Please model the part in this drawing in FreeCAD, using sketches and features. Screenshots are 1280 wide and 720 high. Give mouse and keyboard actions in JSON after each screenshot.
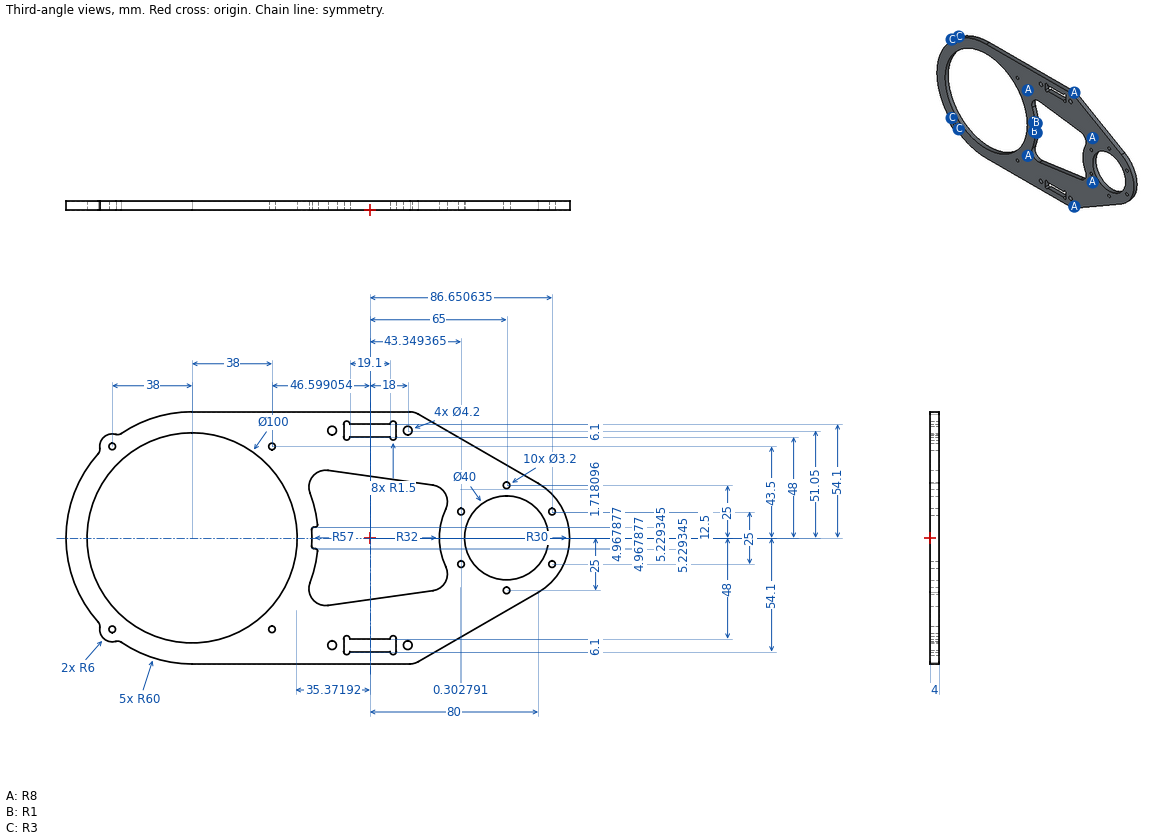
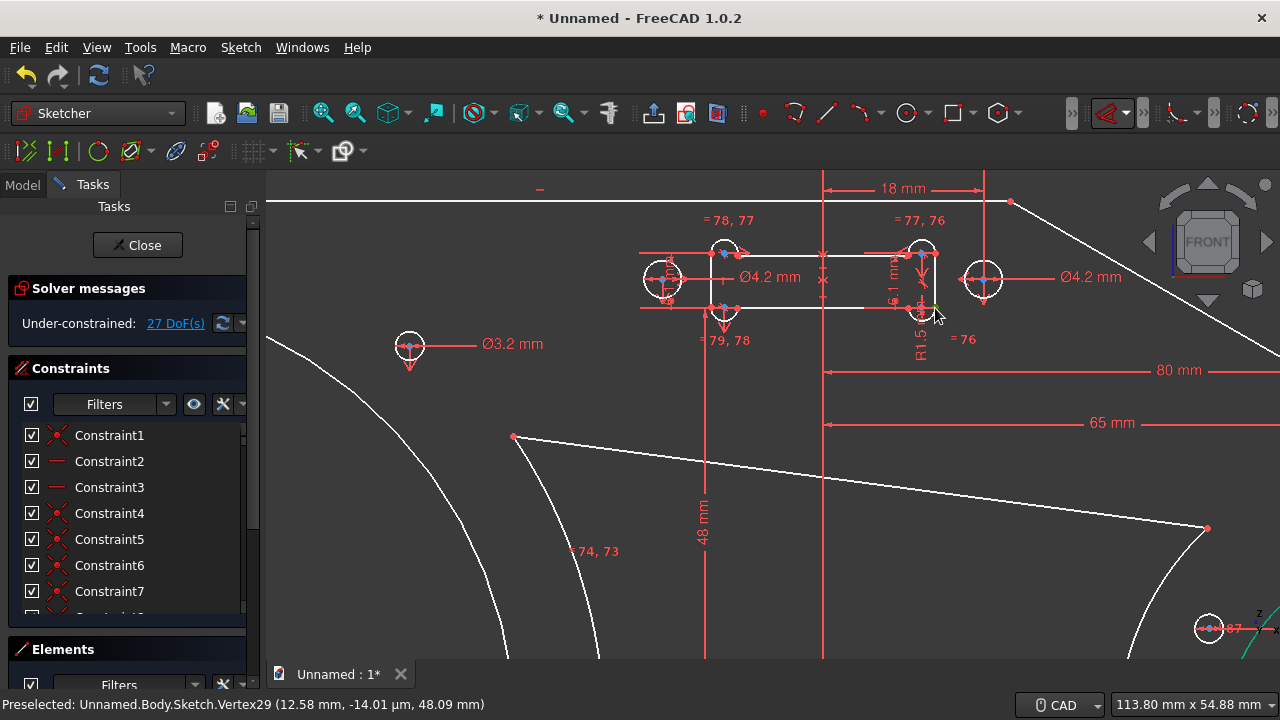
{"action": "left_click", "coordinate": [1128, 114]}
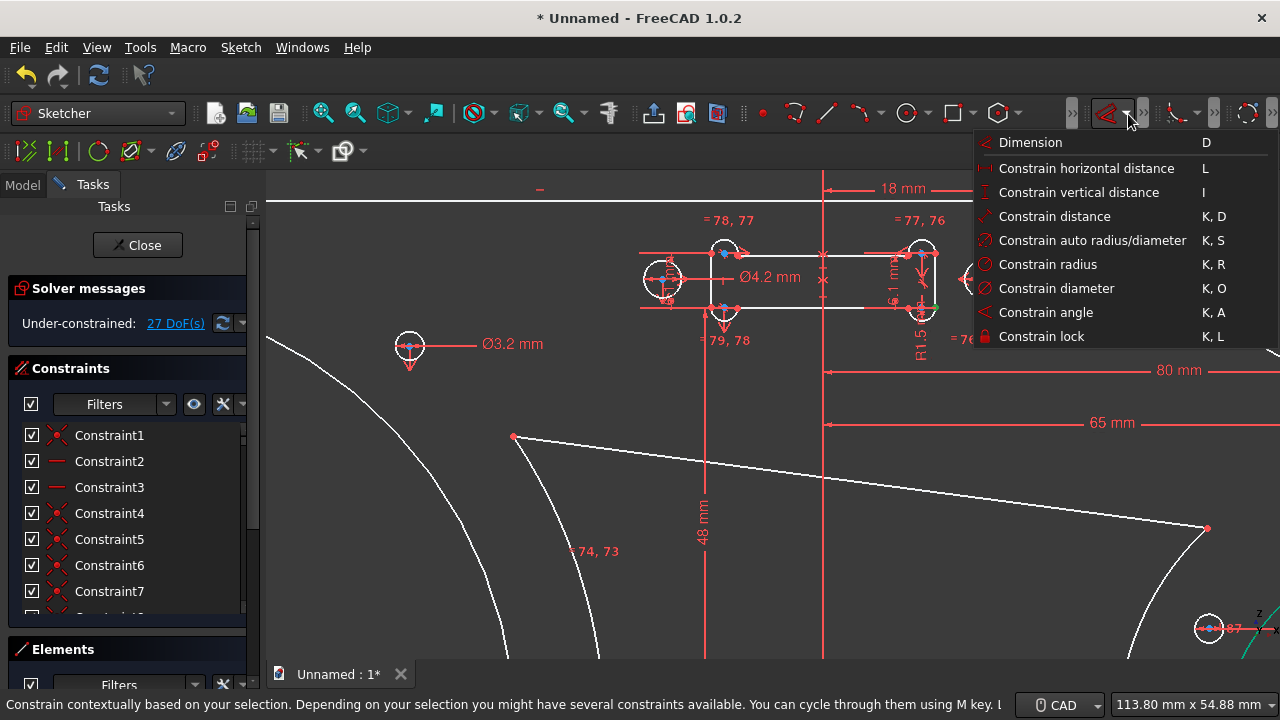
{"action": "left_click", "coordinate": [1126, 192]}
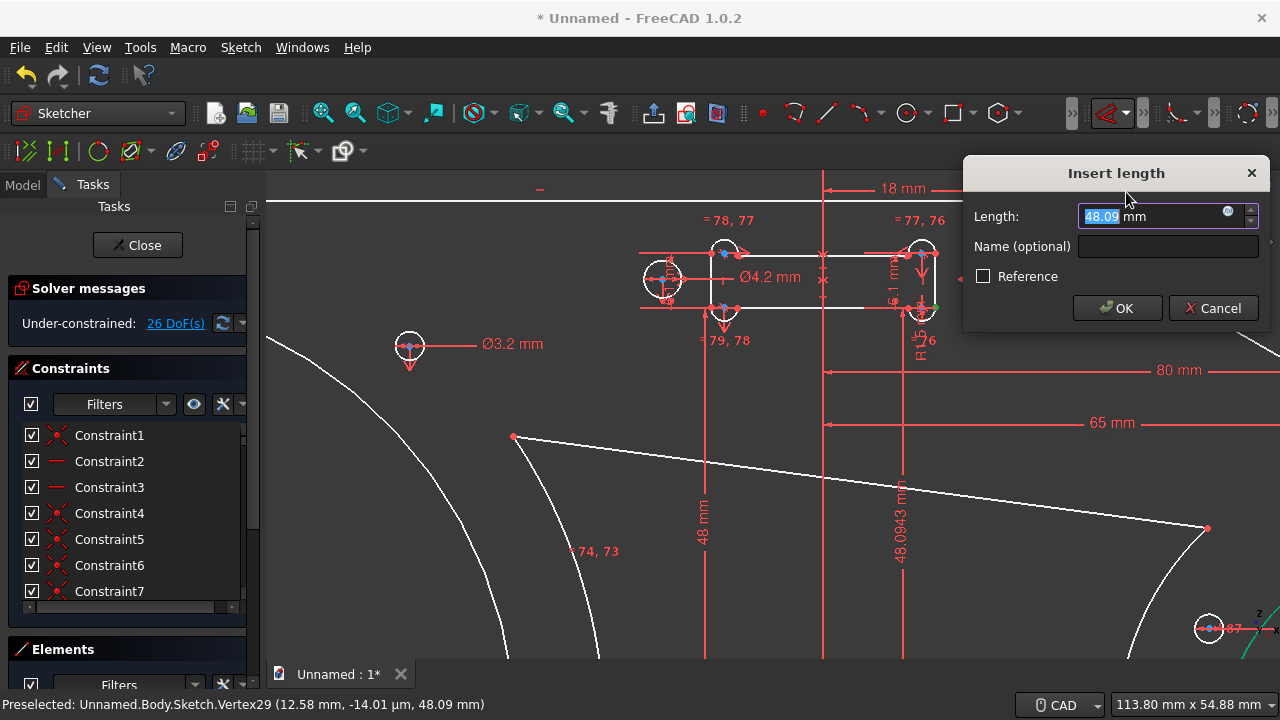
{"action": "type", "text": "48"}
{"action": "key", "text": "Return"}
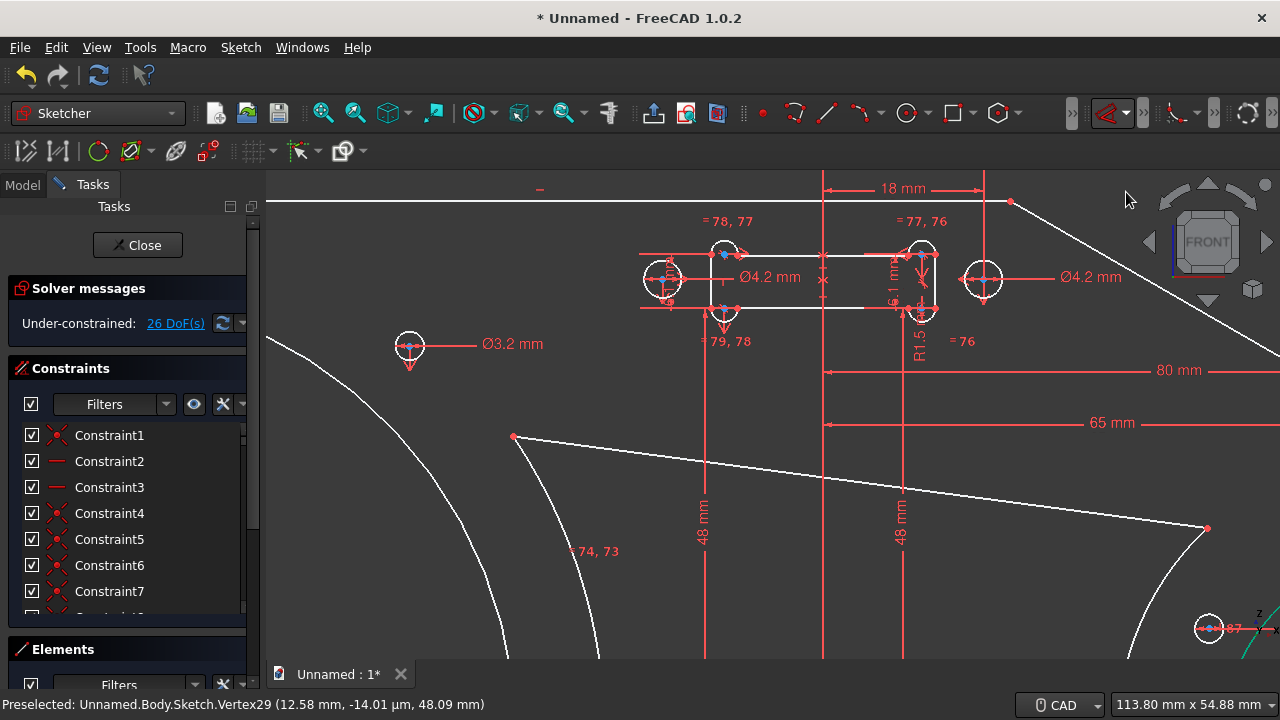
{"action": "scroll", "coordinate": [738, 309], "scroll_direction": "down", "scroll_amount": 7}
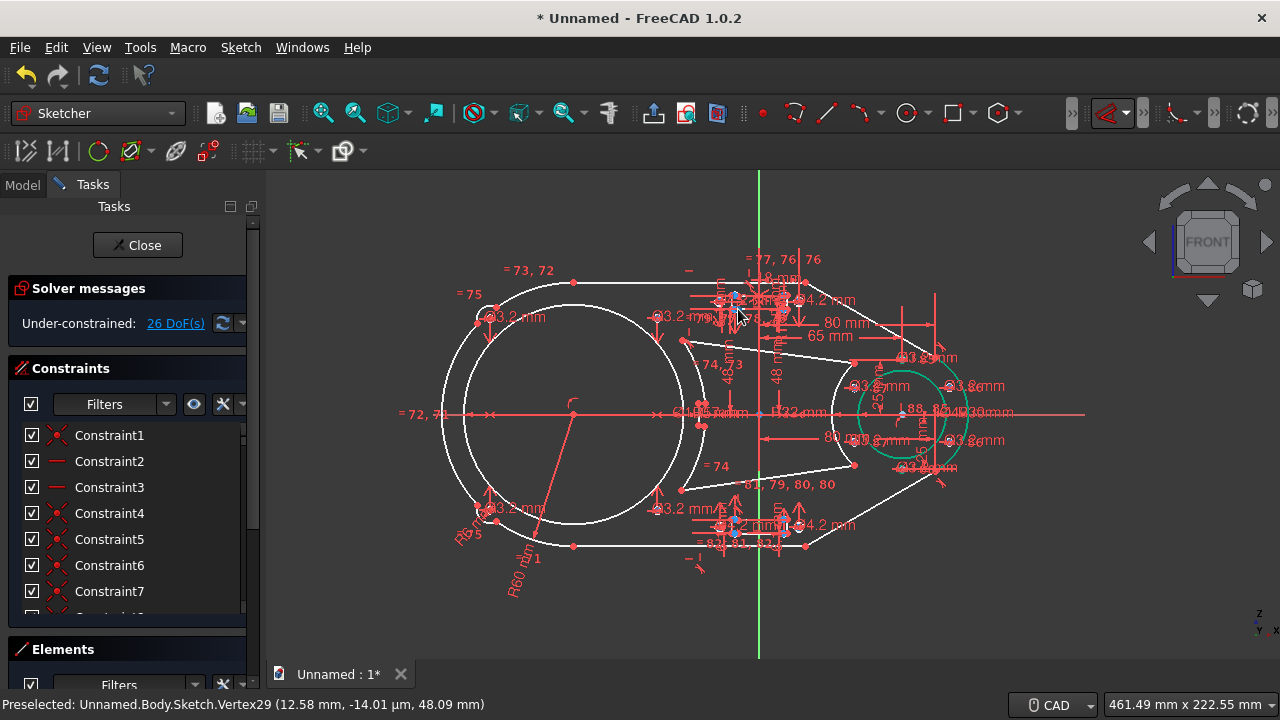
{"action": "scroll", "coordinate": [780, 520], "scroll_direction": "up", "scroll_amount": 7}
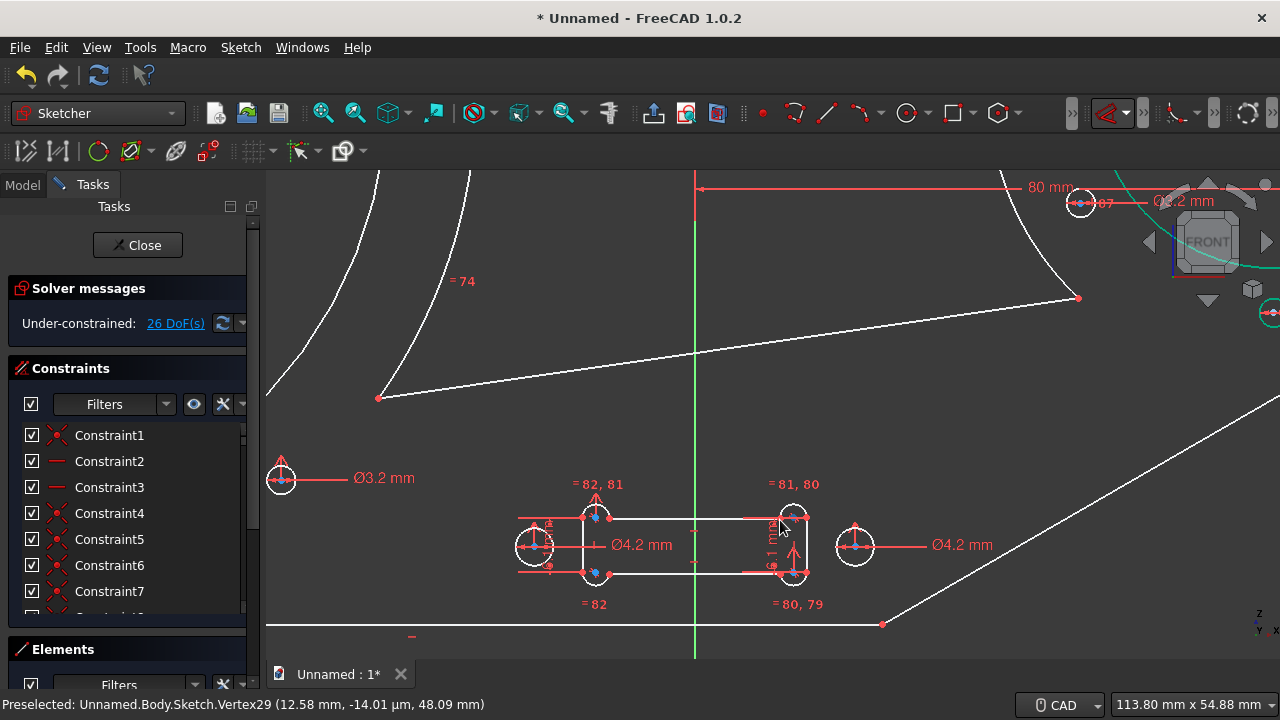
{"action": "left_click", "coordinate": [780, 519]}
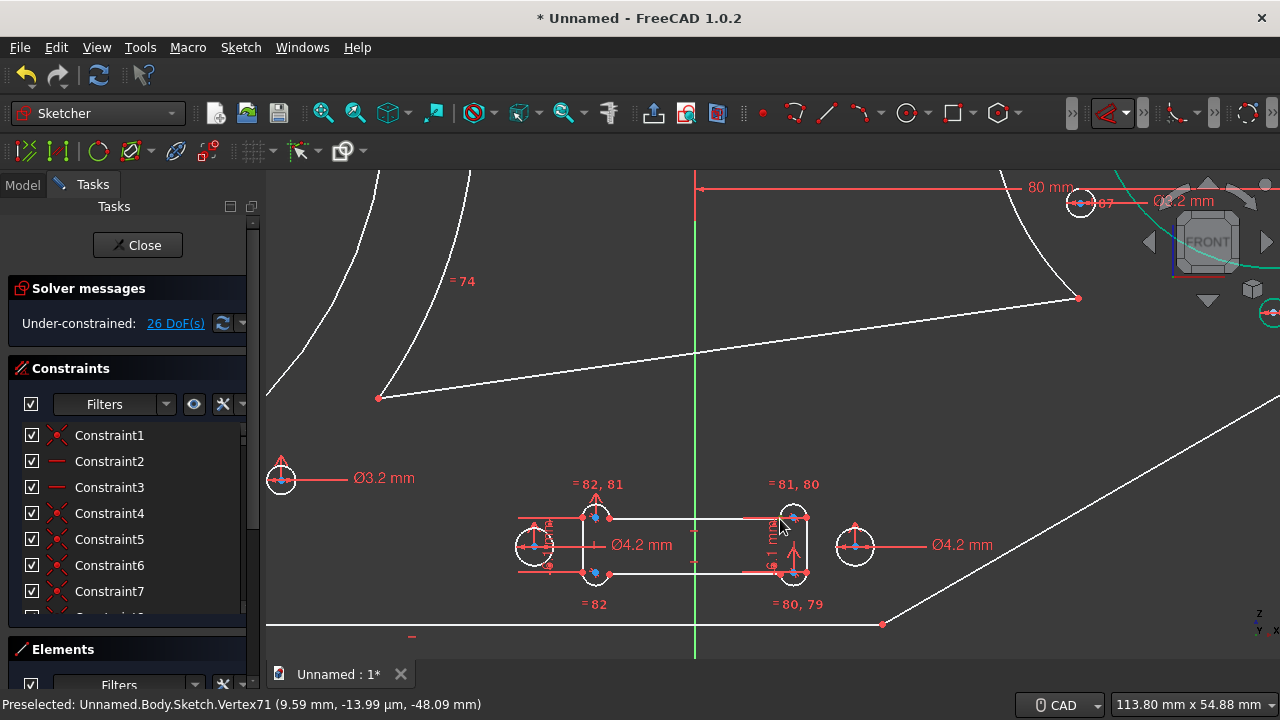
{"action": "key", "text": "i"}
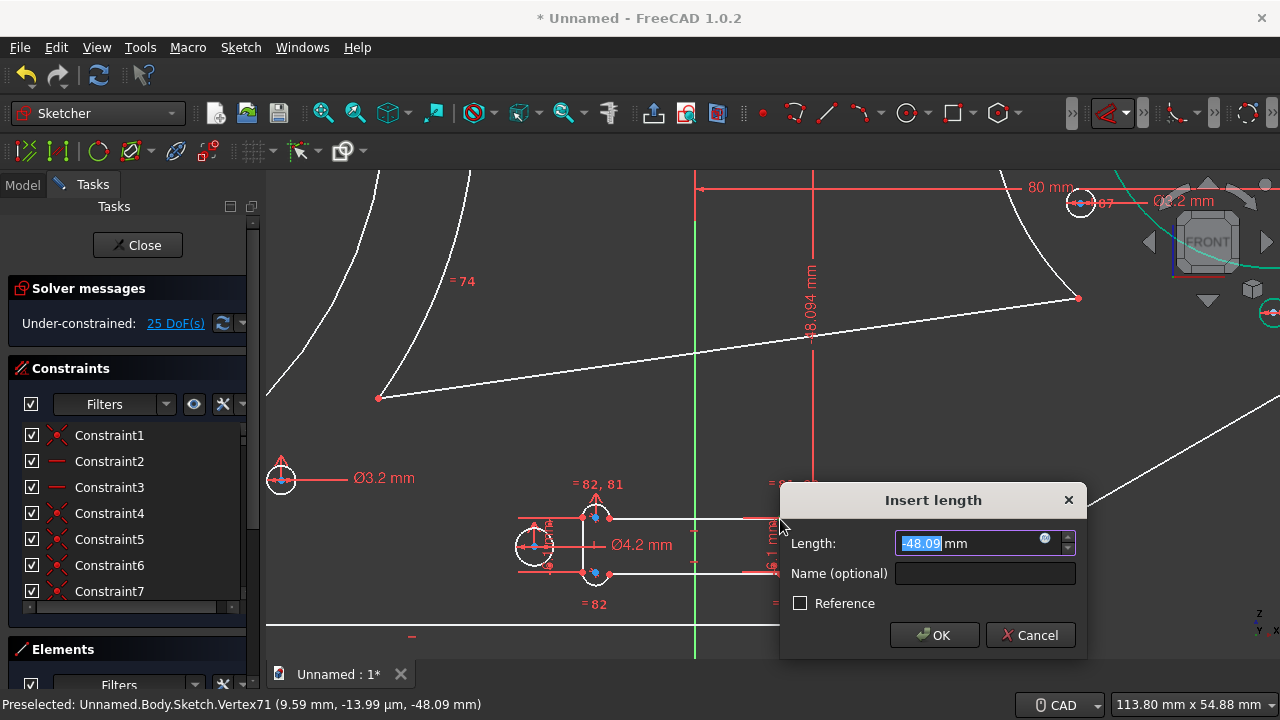
{"action": "type", "text": "-48"}
{"action": "key", "text": "Return"}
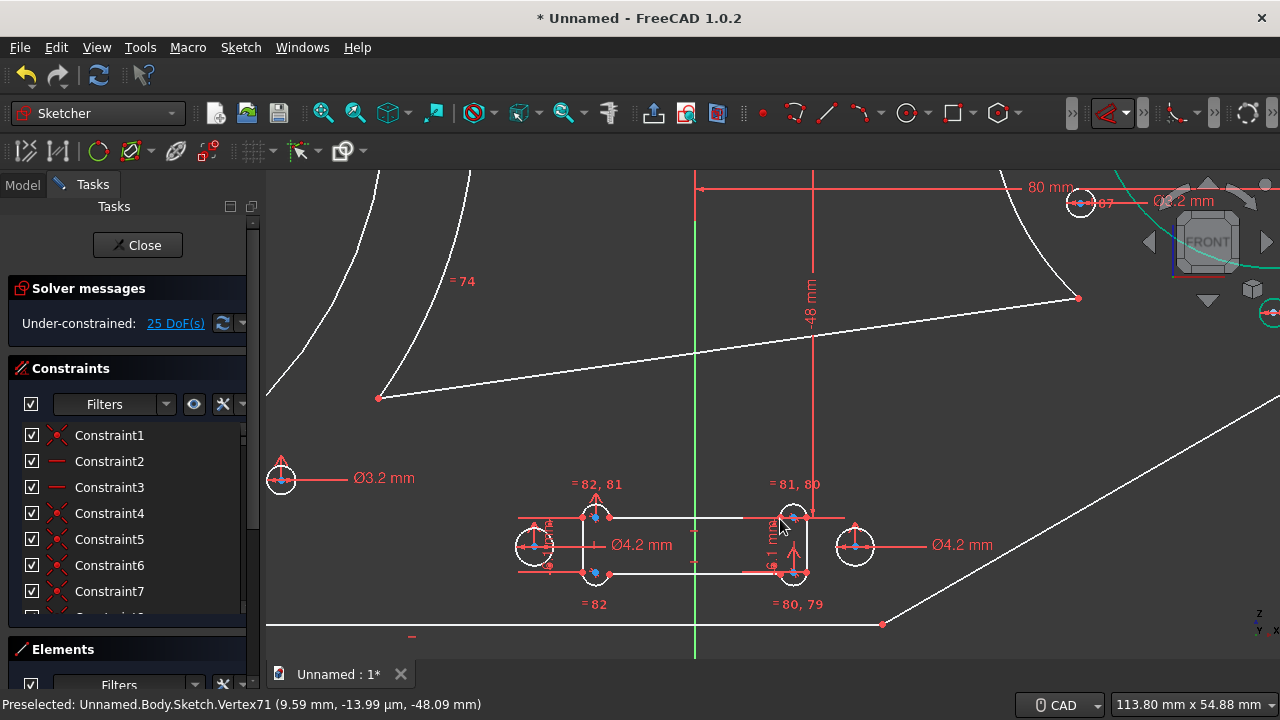
{"action": "scroll", "coordinate": [780, 521], "scroll_direction": "down", "scroll_amount": 7}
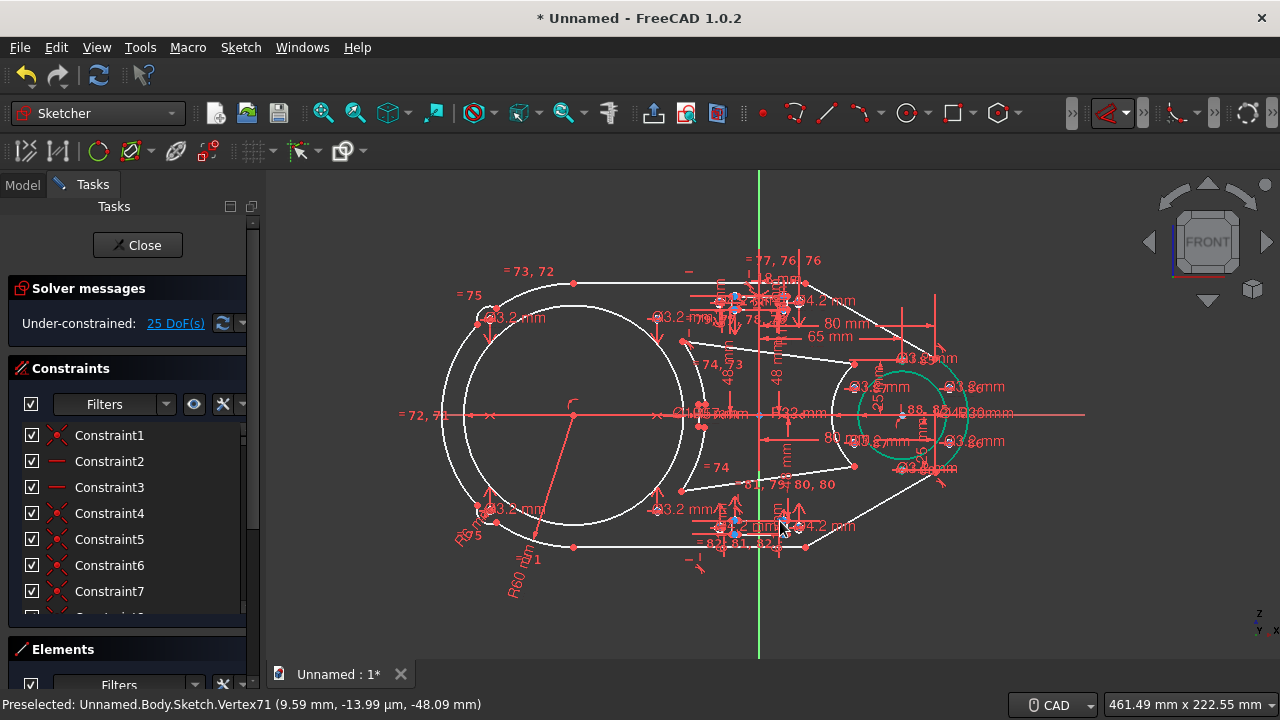
{"action": "left_click", "coordinate": [574, 283]}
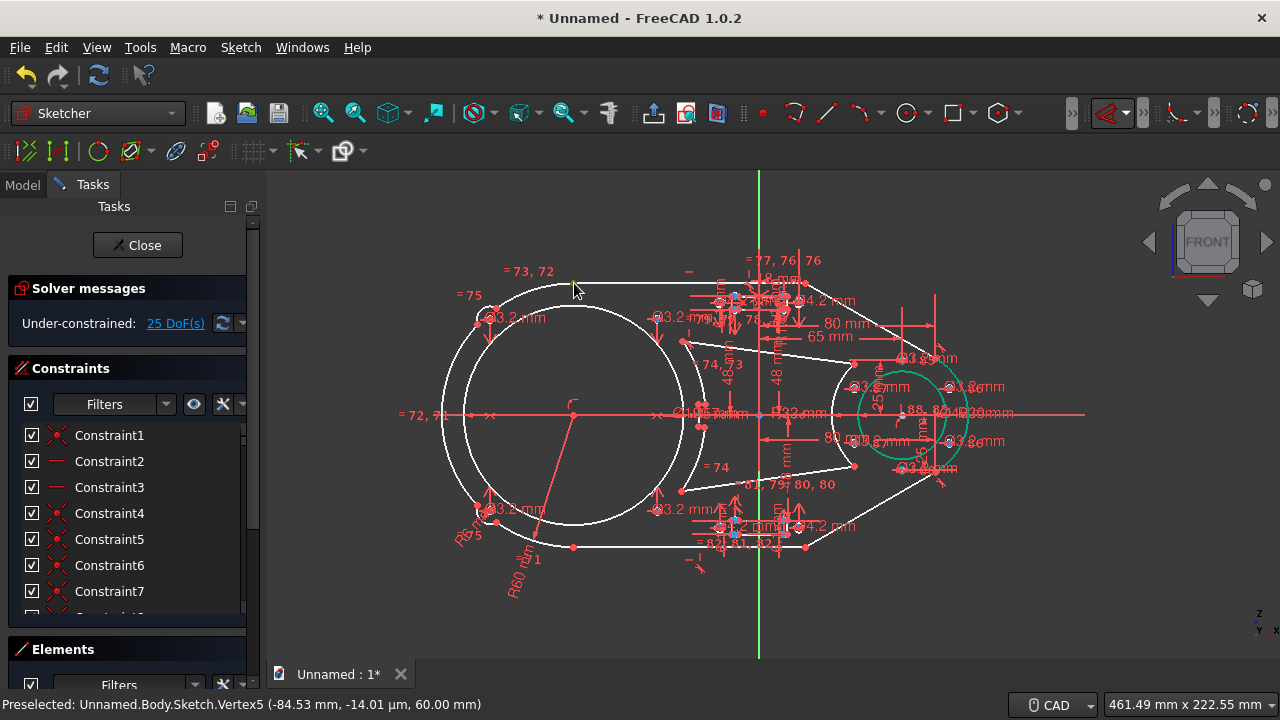
{"action": "left_click", "coordinate": [490, 320]}